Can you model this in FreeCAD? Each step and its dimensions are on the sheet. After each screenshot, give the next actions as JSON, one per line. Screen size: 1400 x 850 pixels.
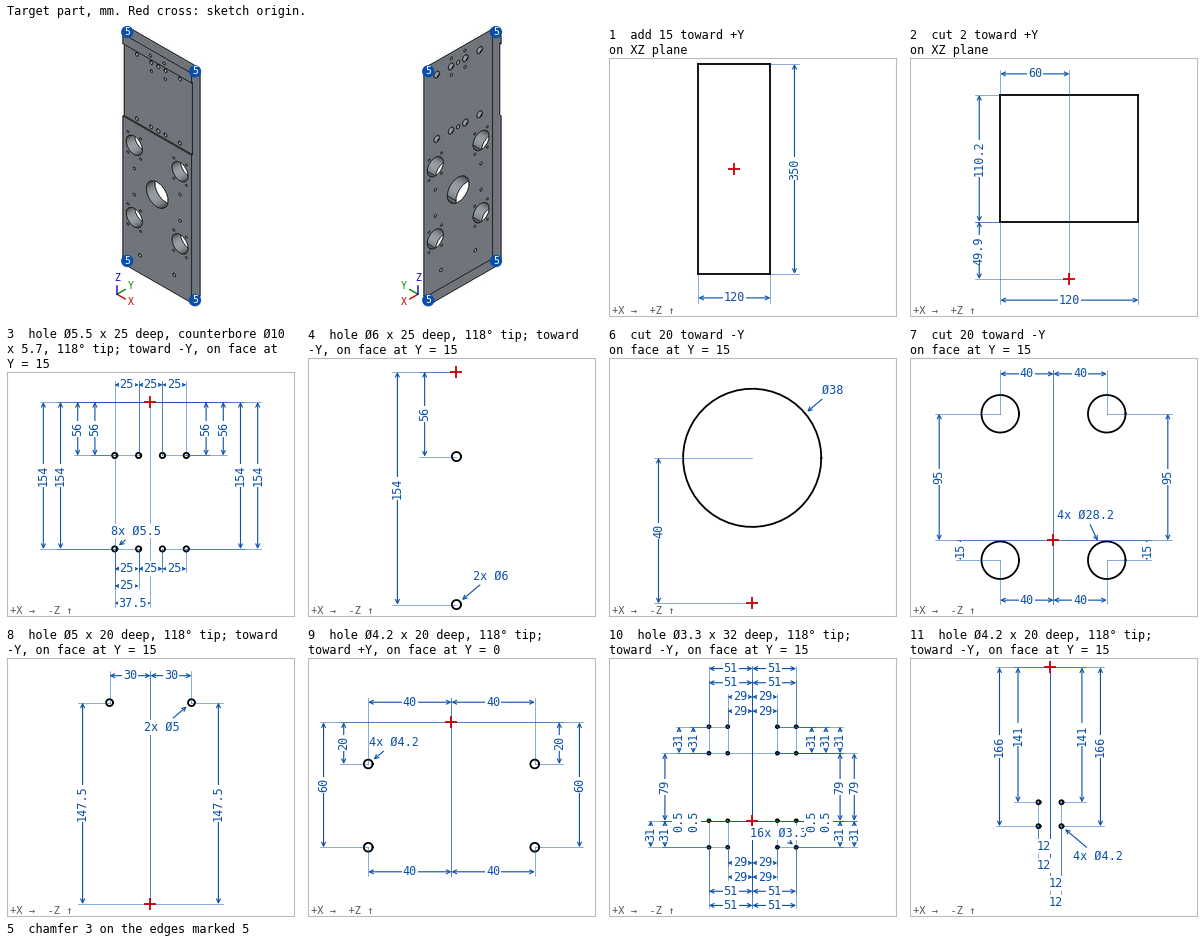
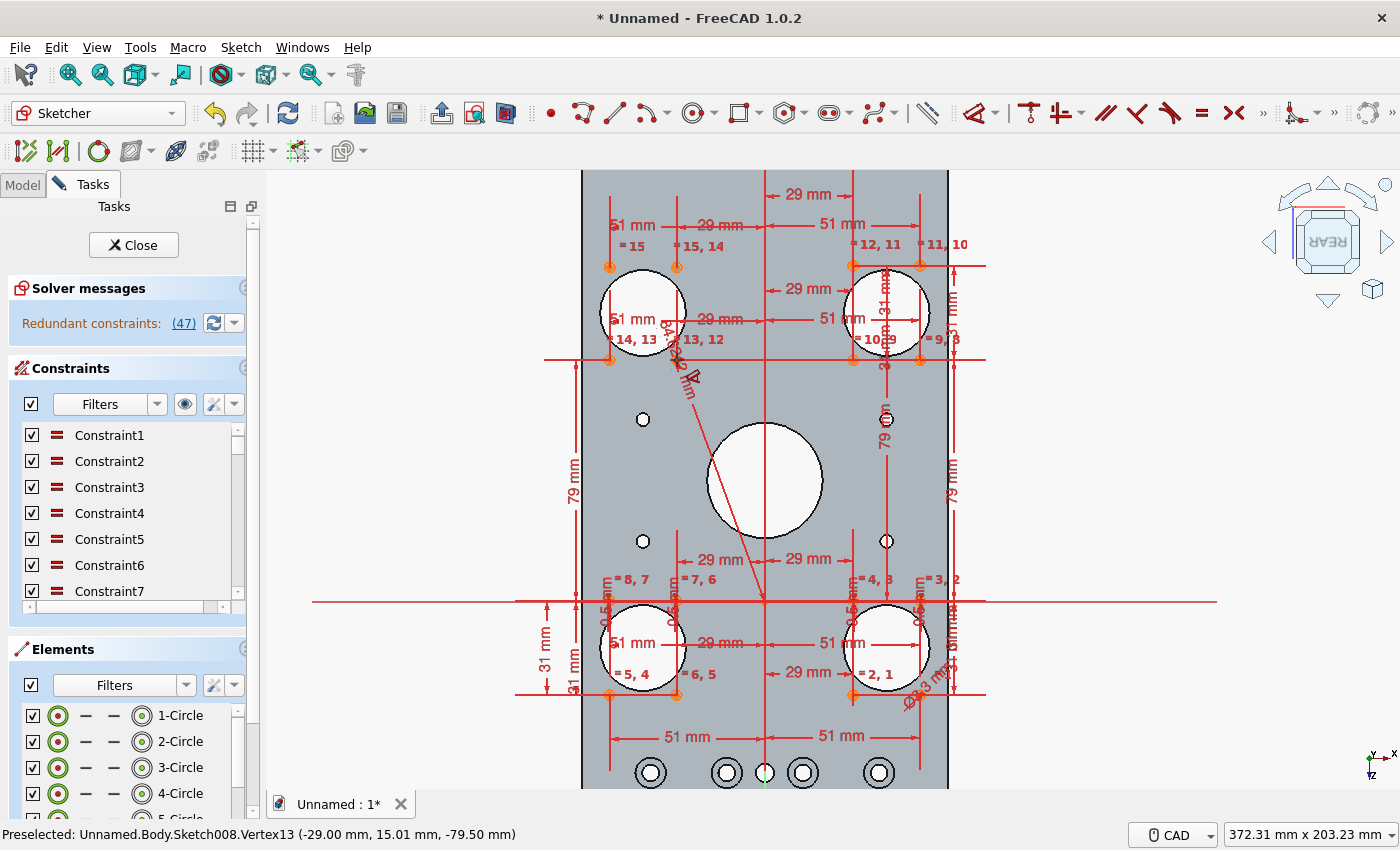
{"action": "left_click", "coordinate": [677, 267]}
{"action": "left_click", "coordinate": [643, 293]}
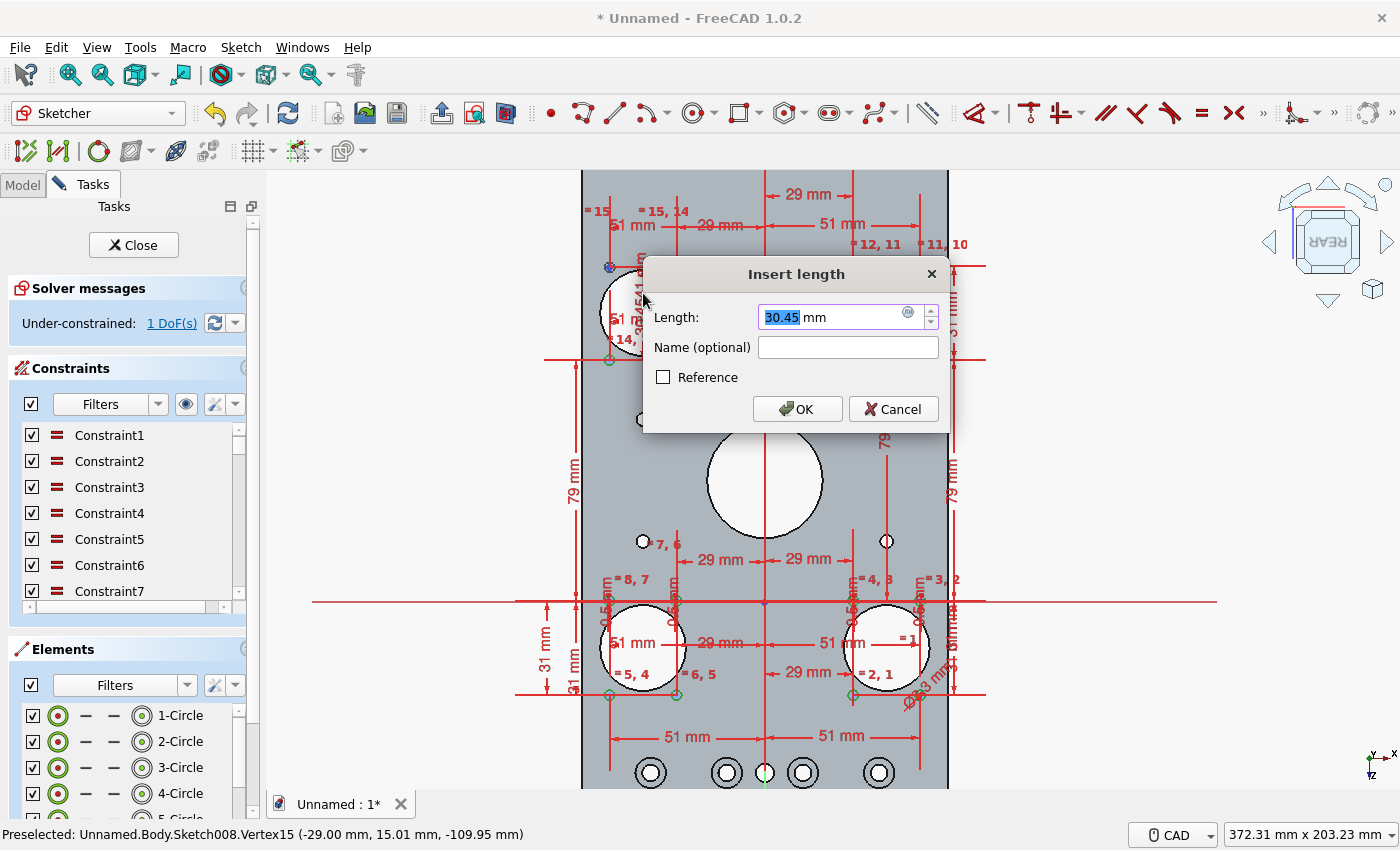
{"action": "type", "text": "31"}
{"action": "key", "text": "Return"}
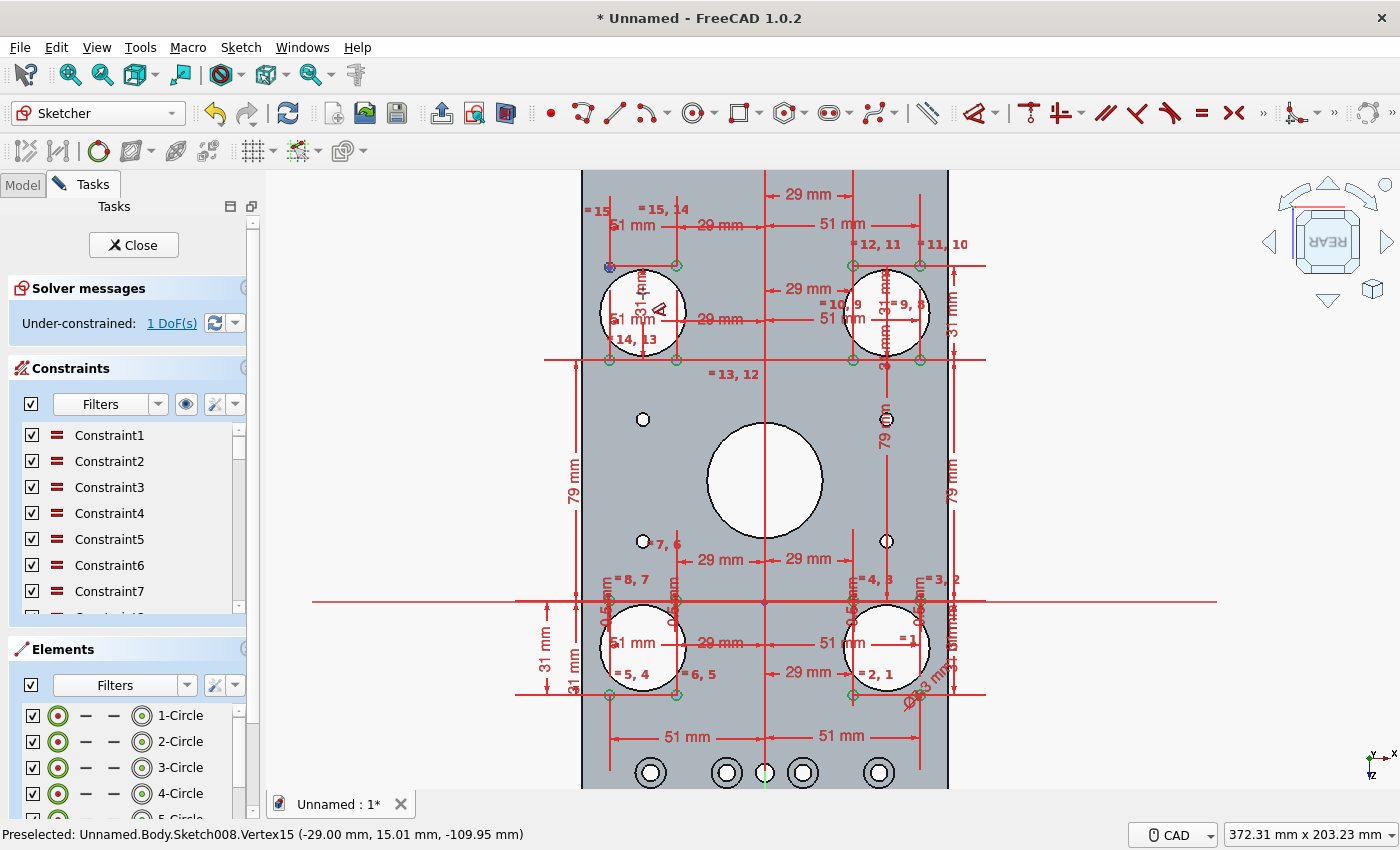
{"action": "left_click", "coordinate": [610, 360]}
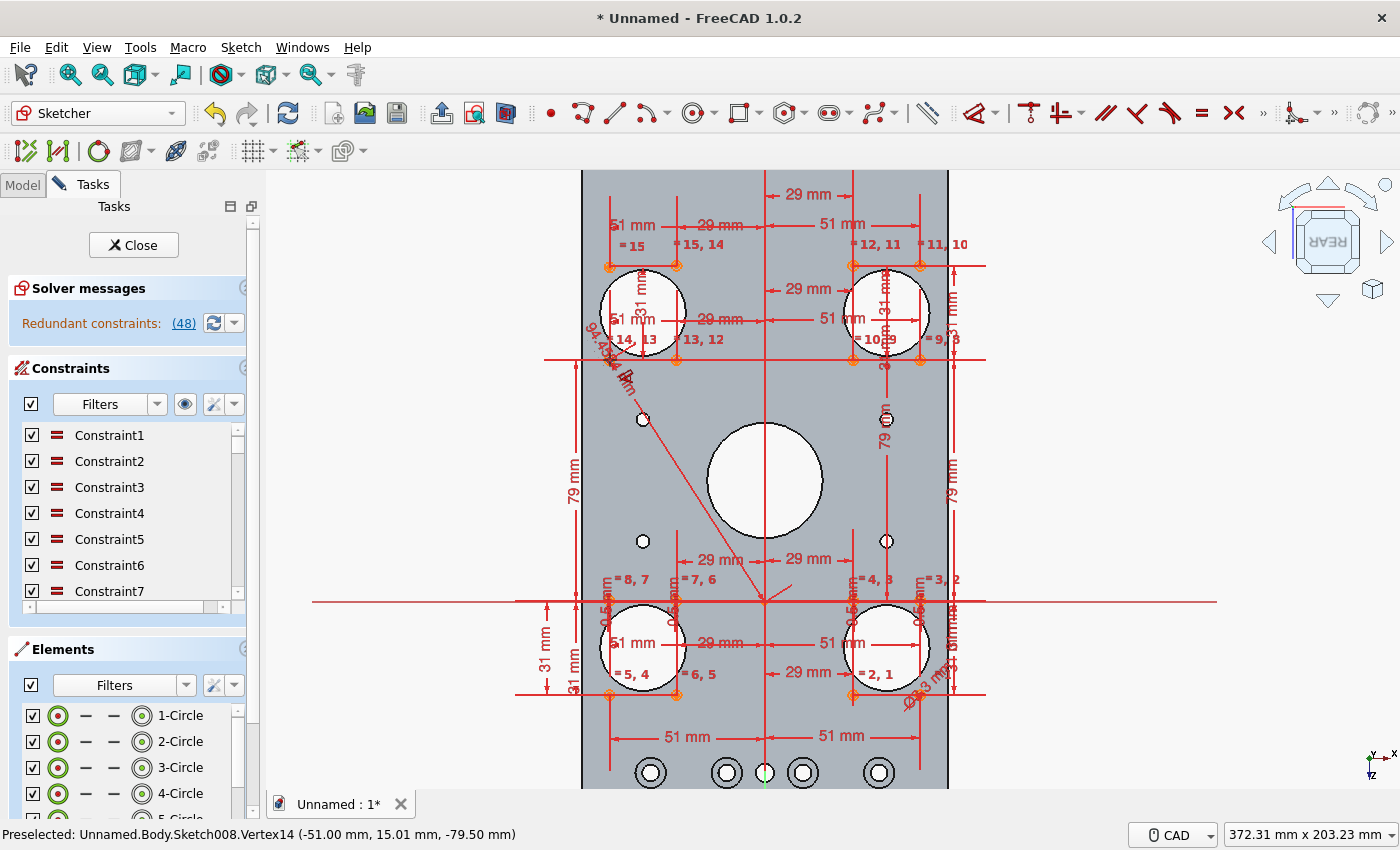
{"action": "left_click", "coordinate": [610, 267]}
{"action": "left_click", "coordinate": [576, 346]}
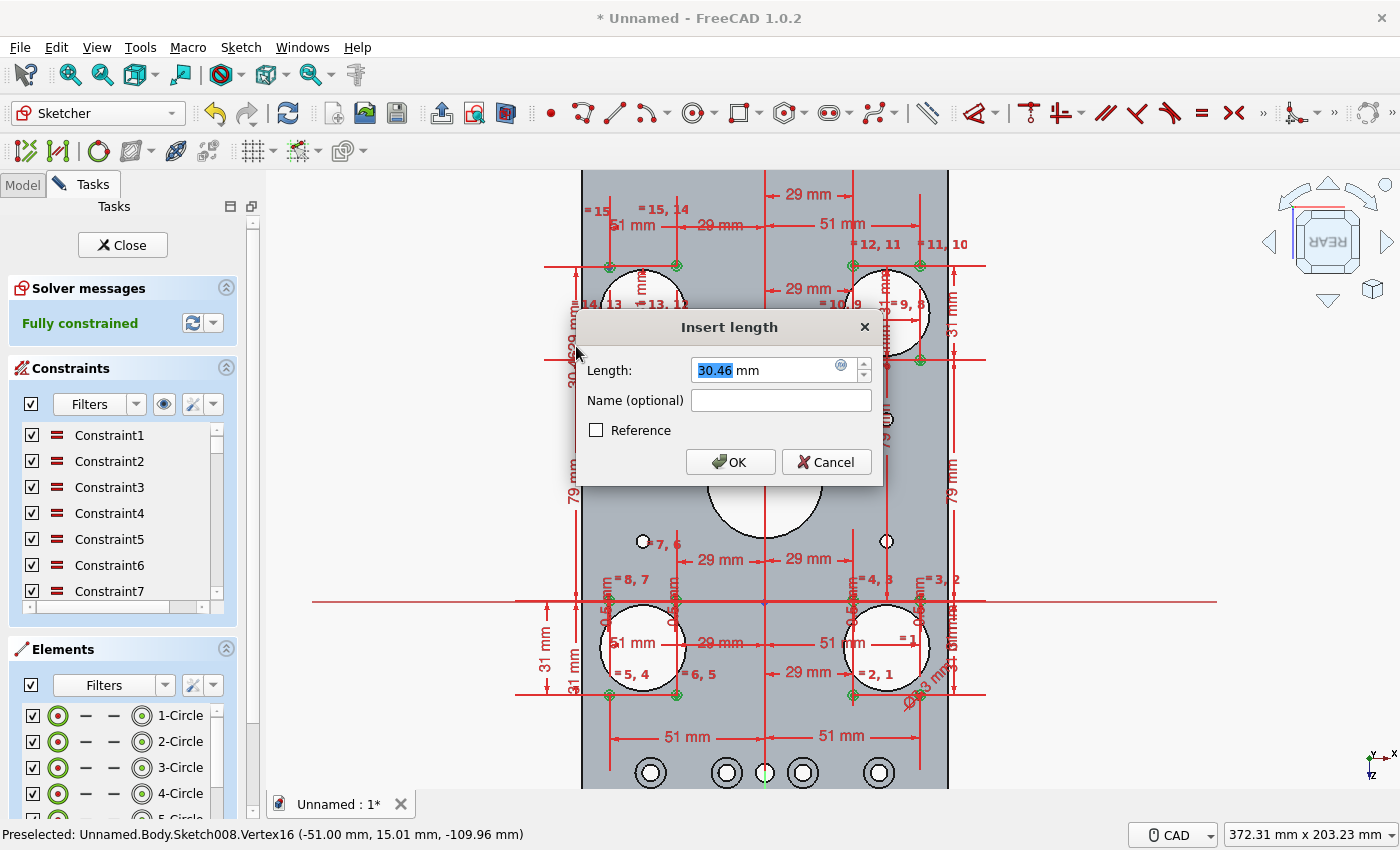
{"action": "type", "text": "31"}
{"action": "key", "text": "Return"}
{"action": "key", "text": "Escape"}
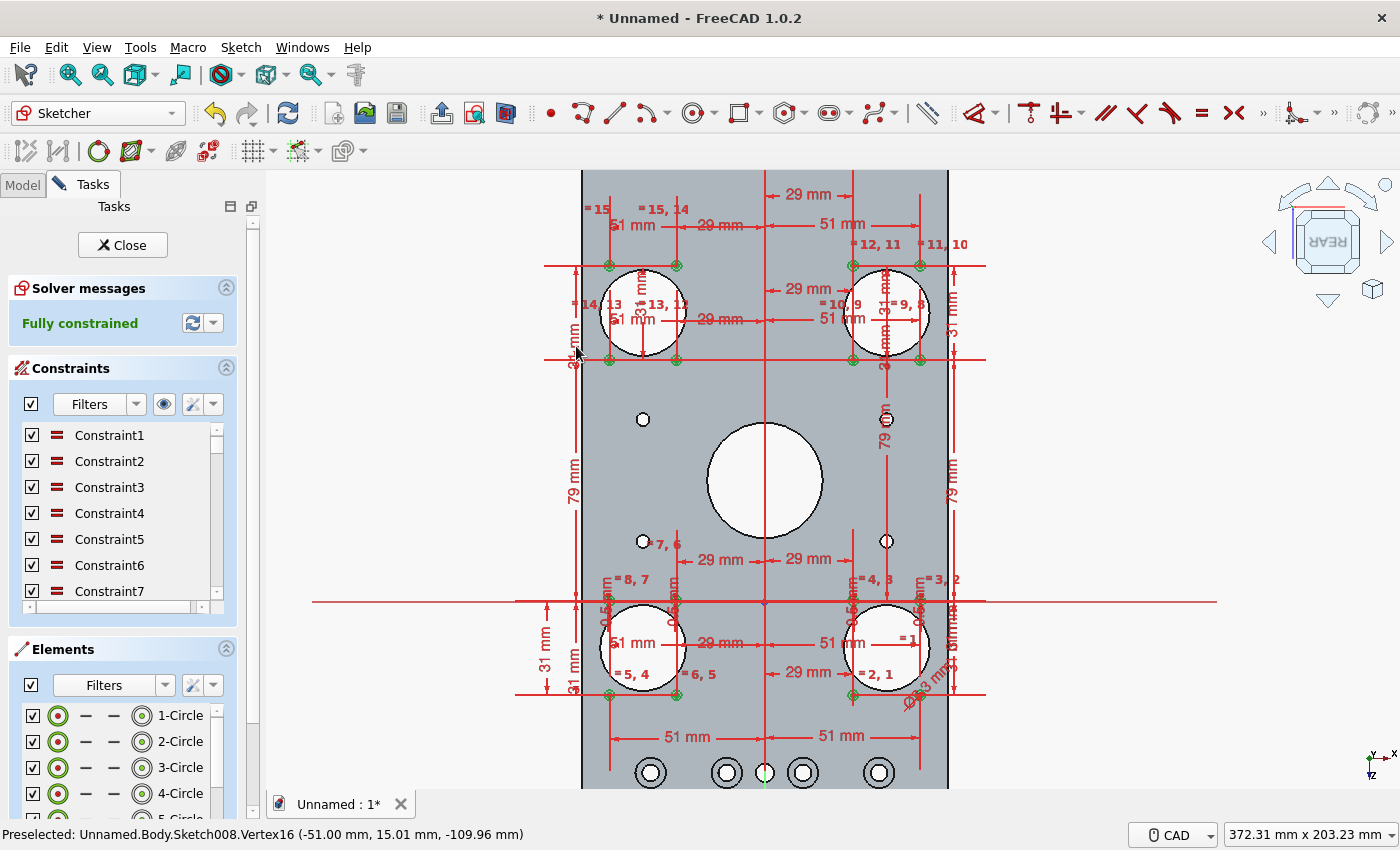
{"action": "left_click", "coordinate": [123, 245]}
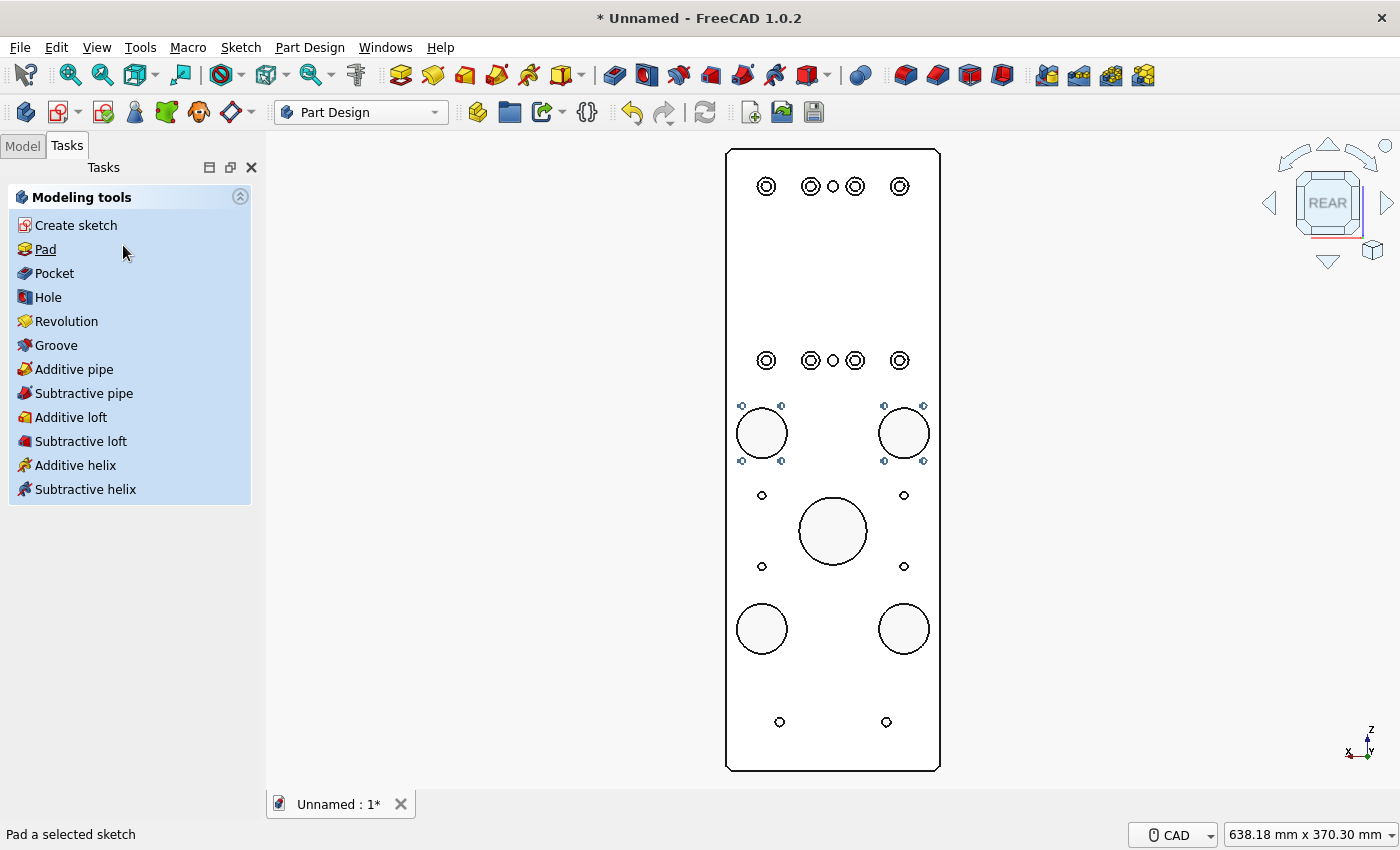
{"action": "left_click", "coordinate": [648, 76]}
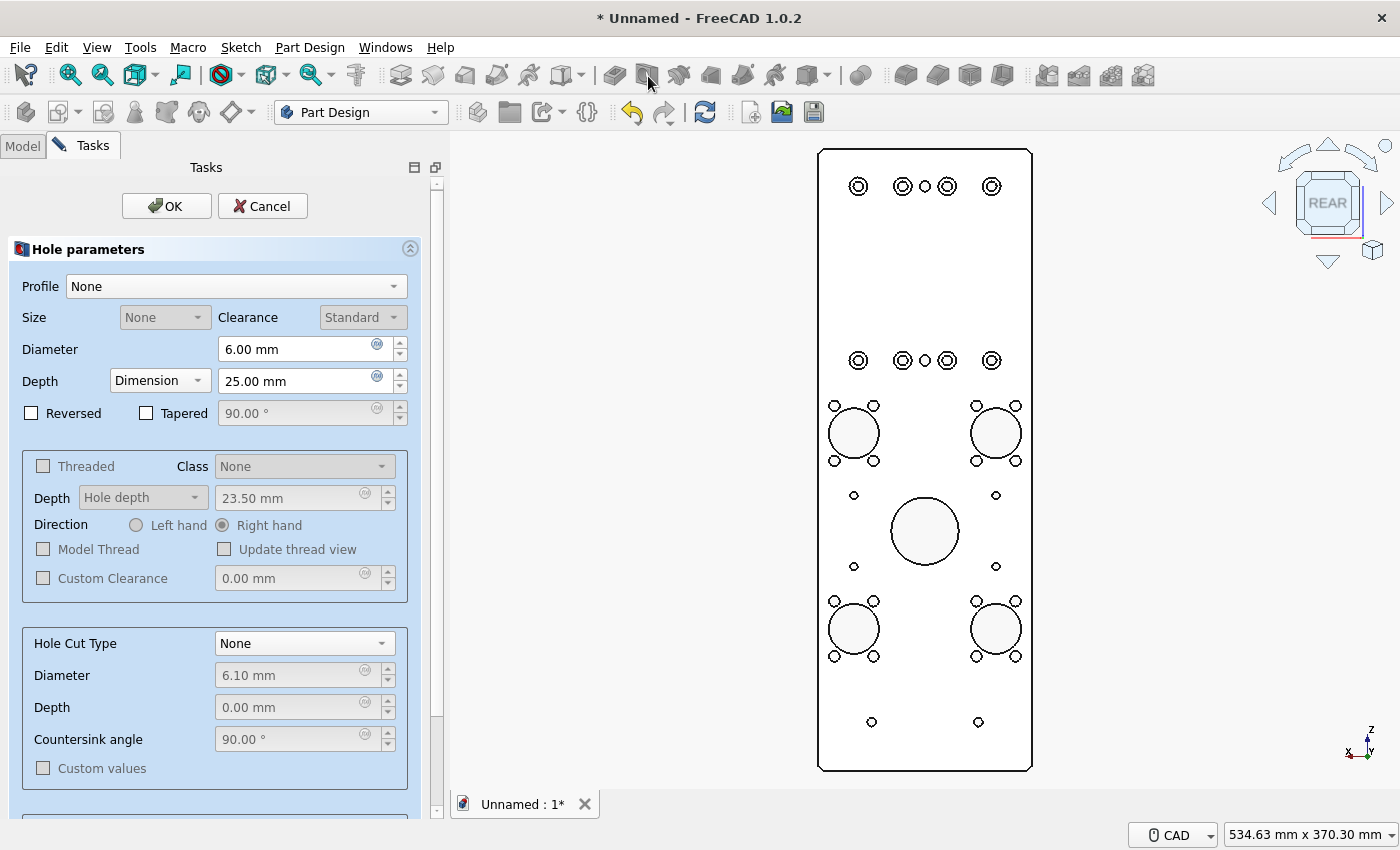
{"action": "triple_click", "coordinate": [305, 349]}